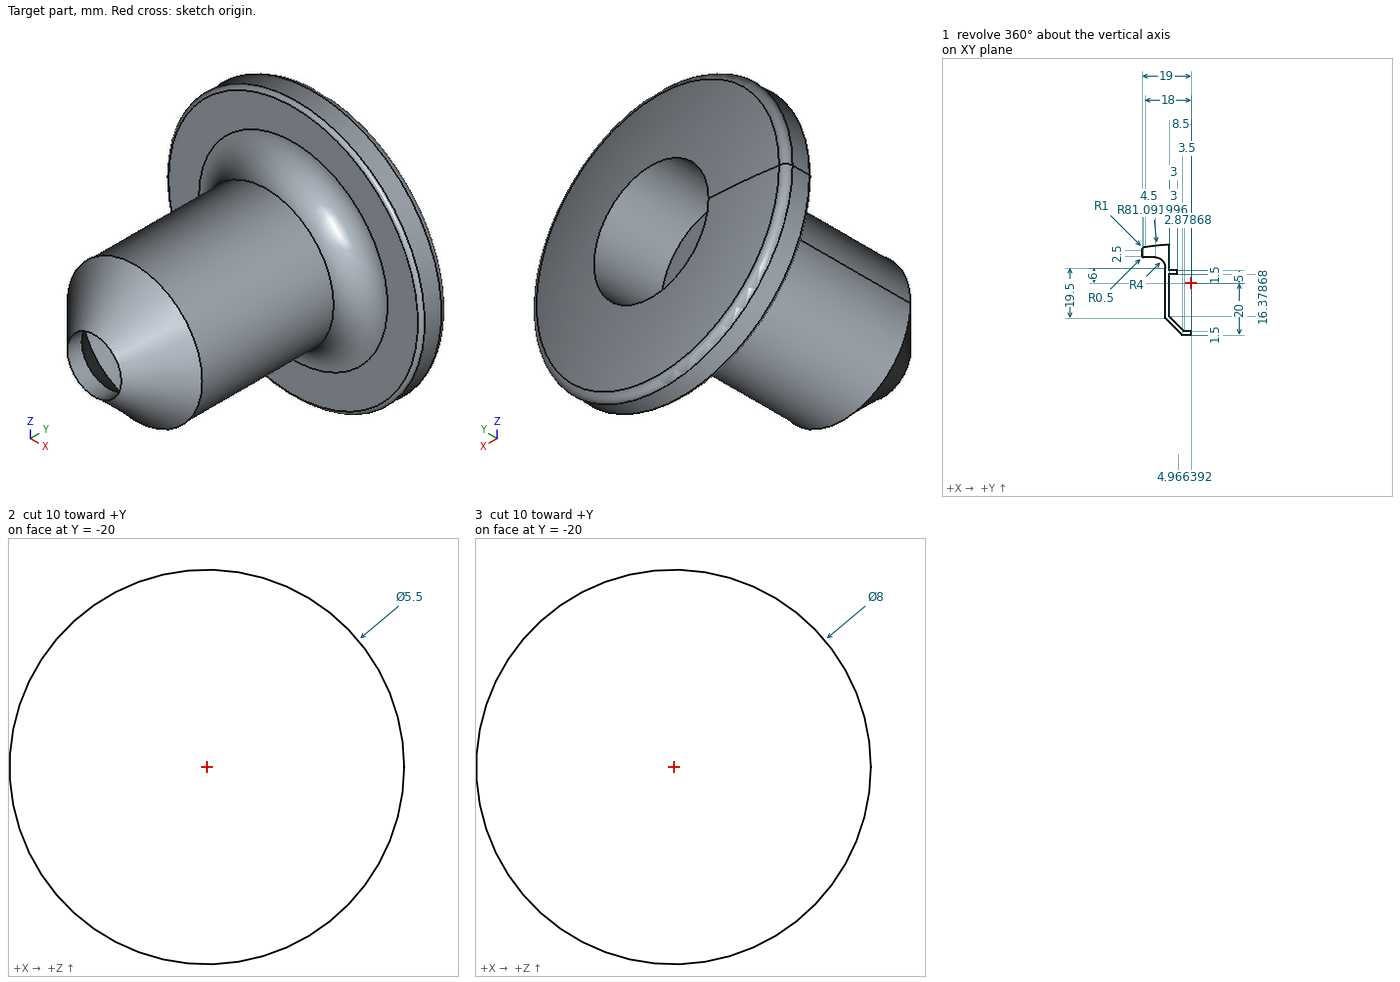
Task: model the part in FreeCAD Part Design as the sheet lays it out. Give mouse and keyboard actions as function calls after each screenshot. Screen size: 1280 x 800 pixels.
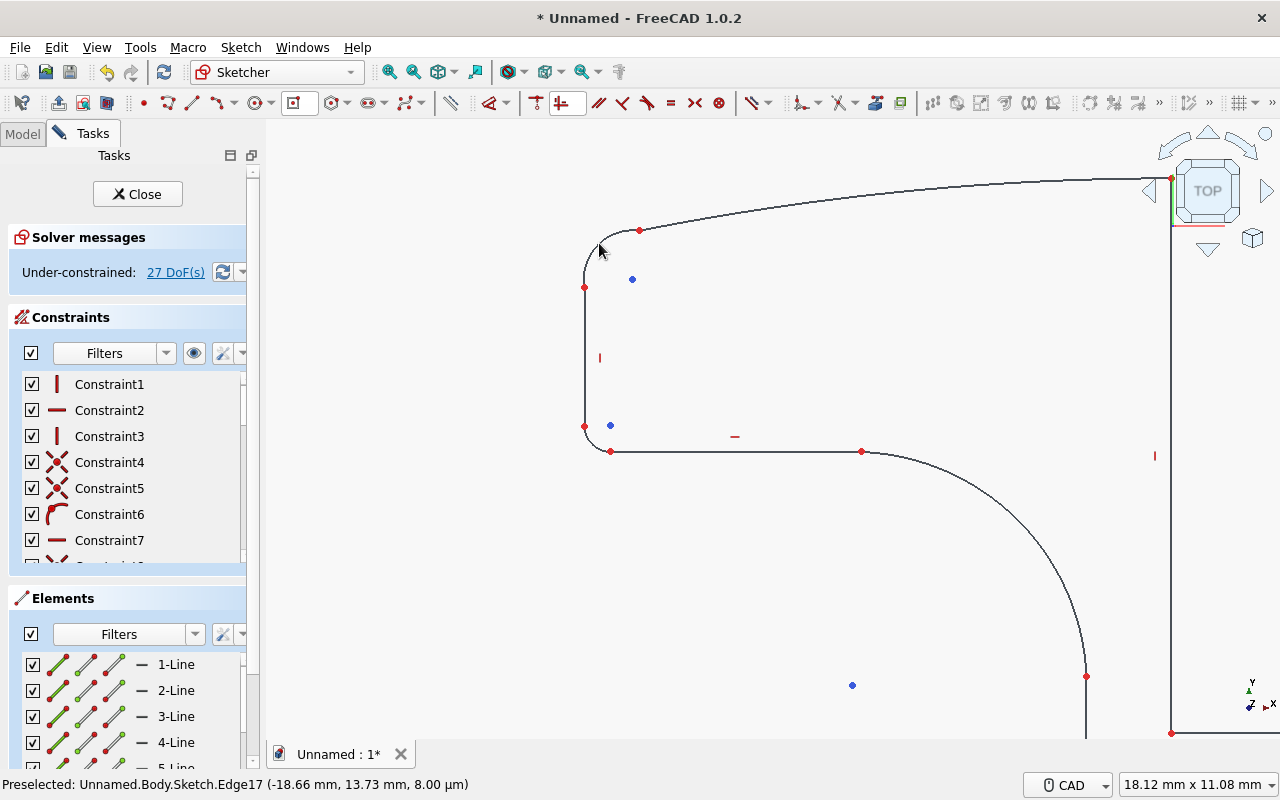
scroll(601, 247, down, 8)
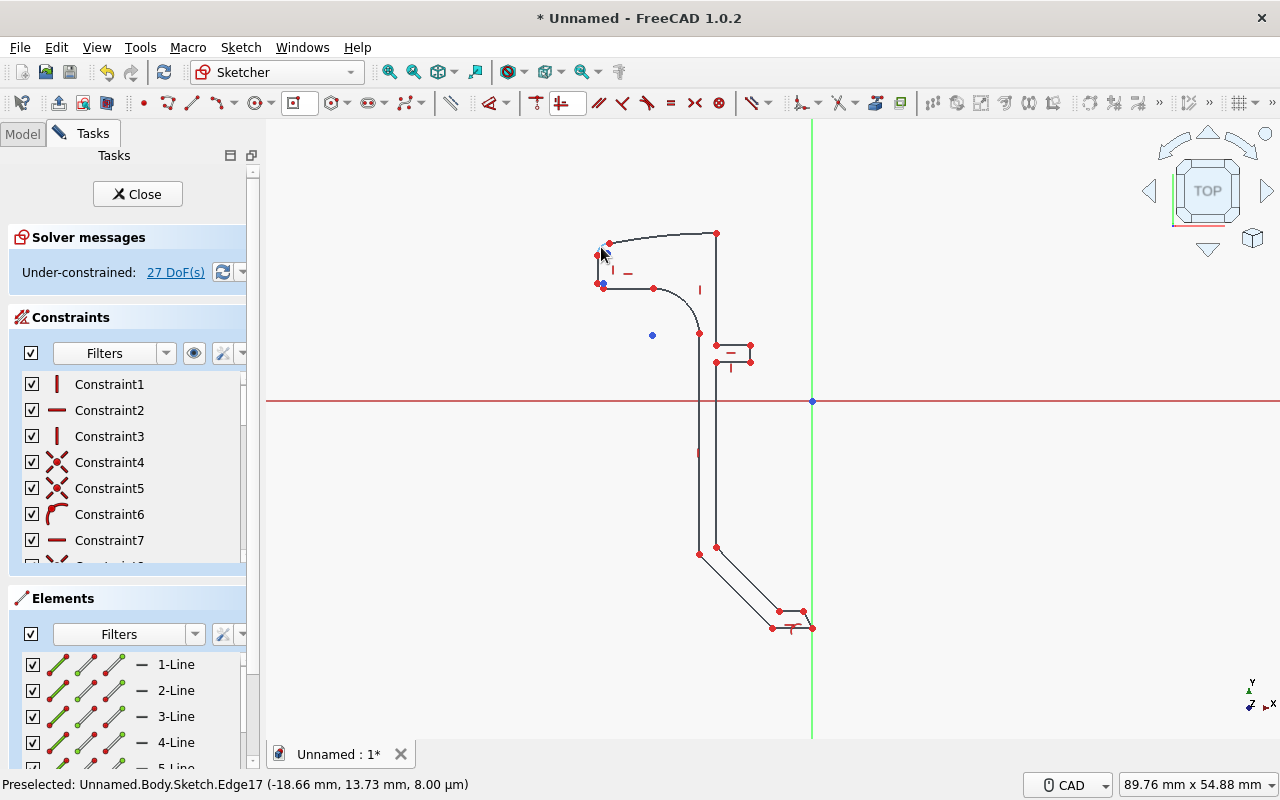
scroll(598, 264, up, 3)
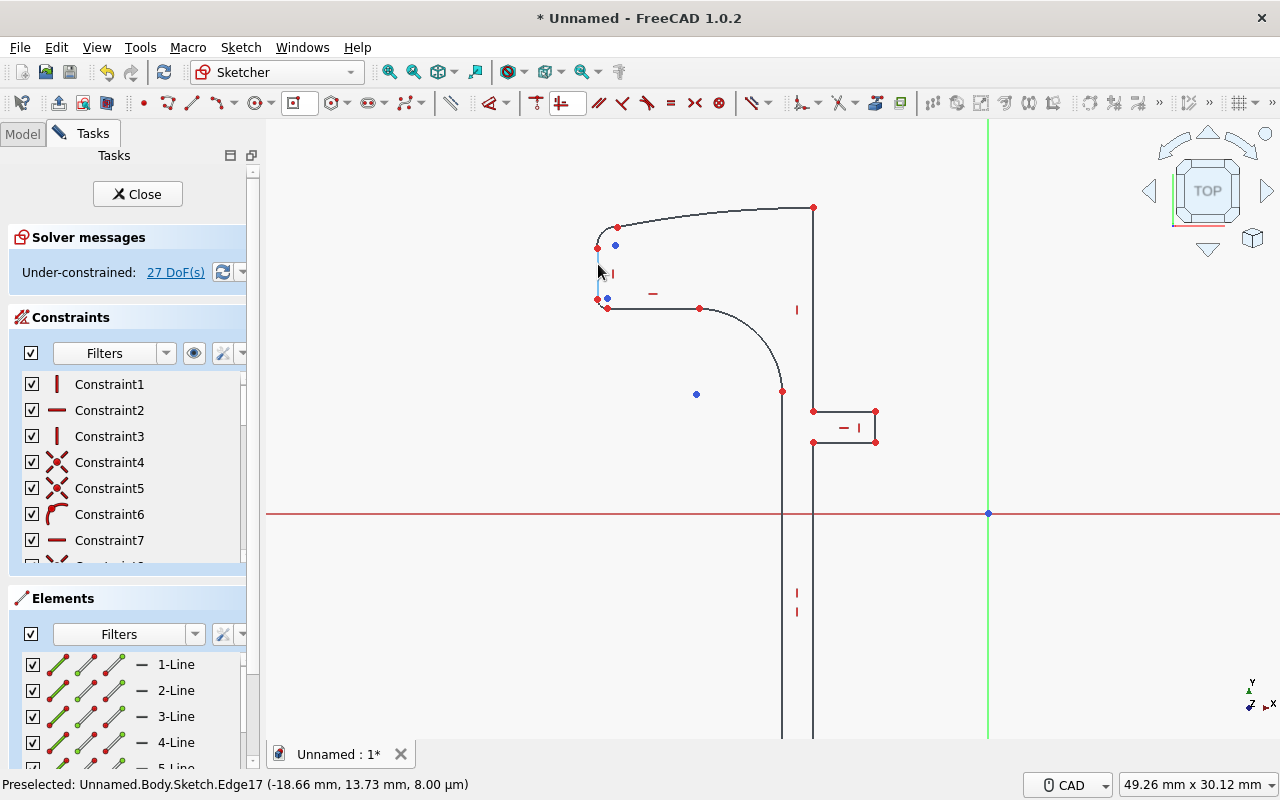
click(598, 263)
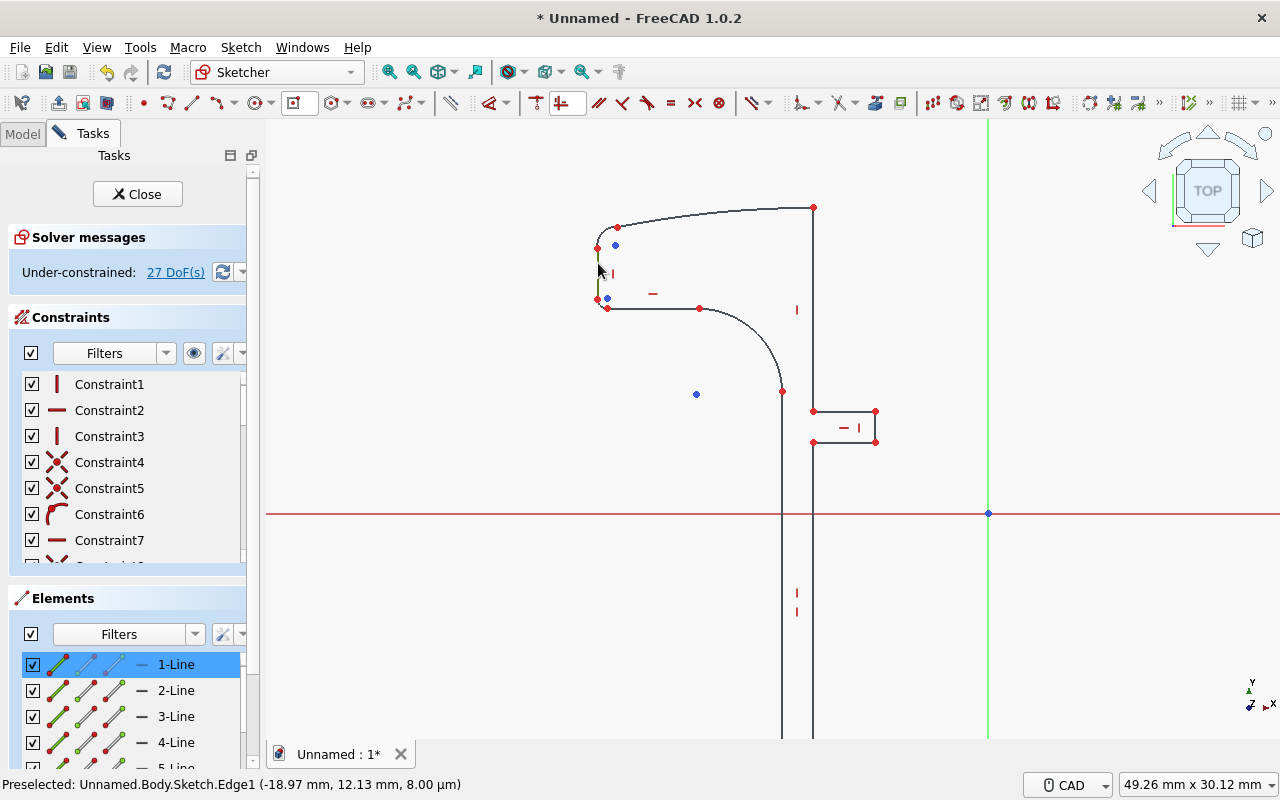
scroll(600, 306, up, 4)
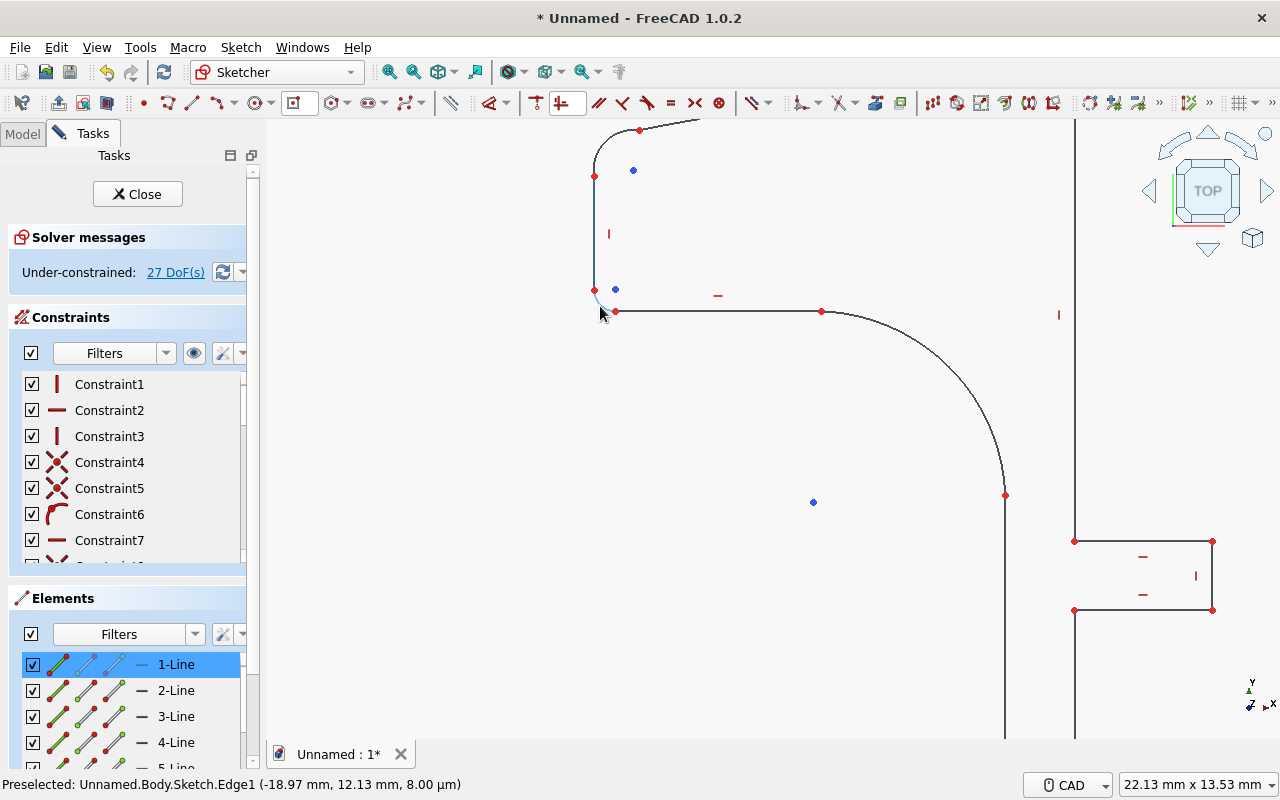
click(601, 305)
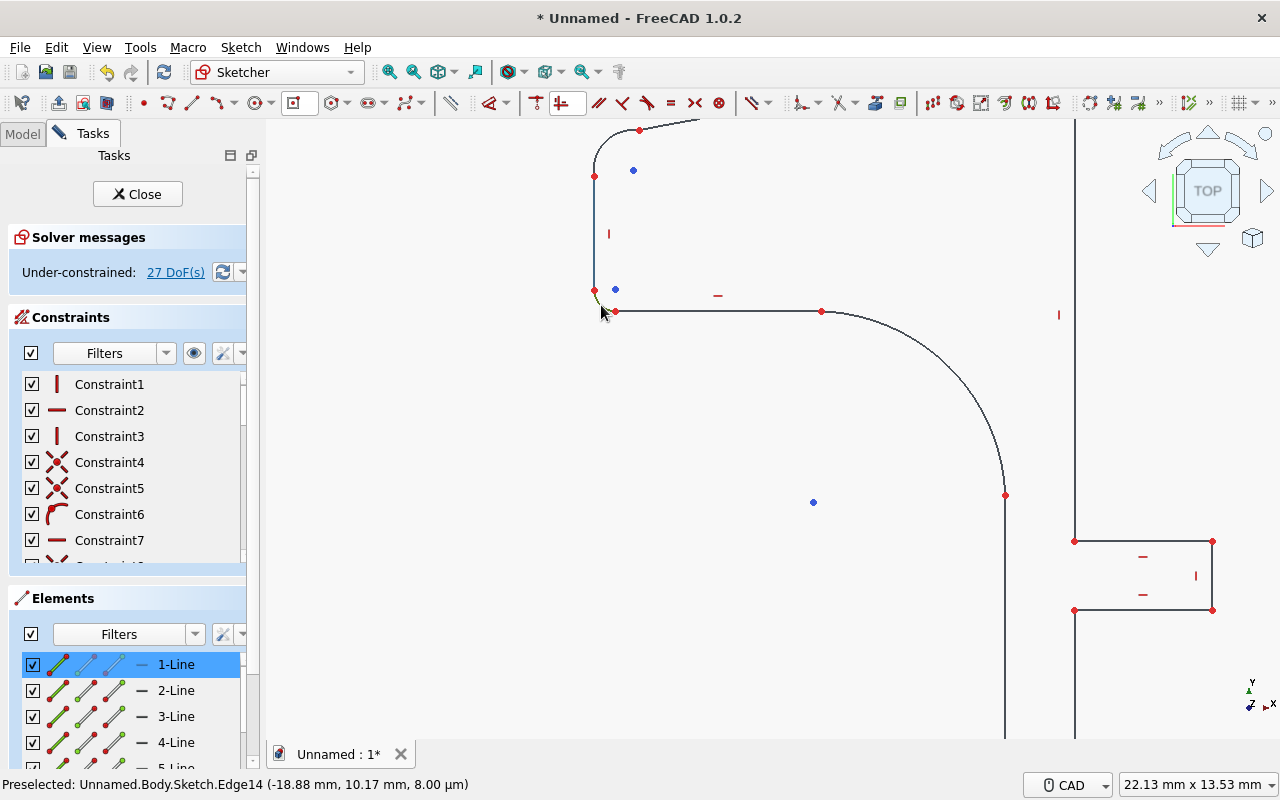
key(t)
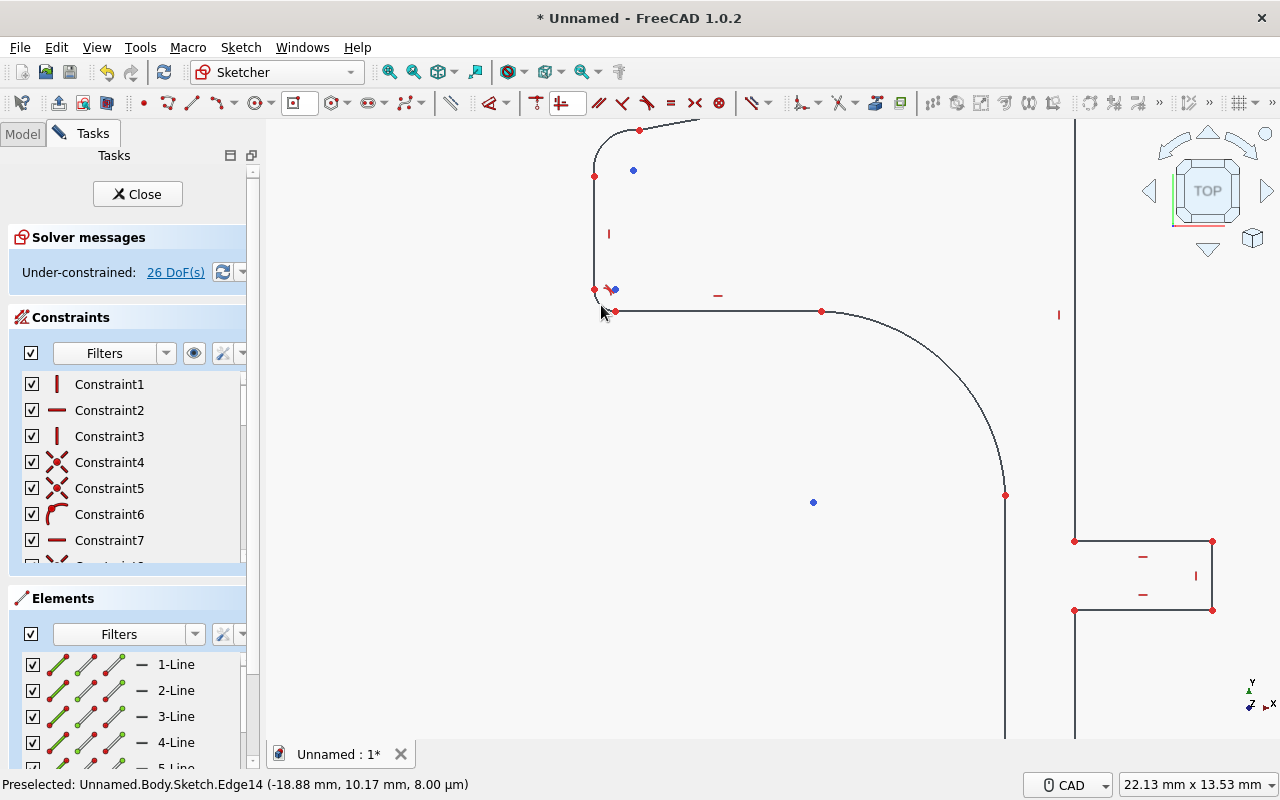
click(594, 211)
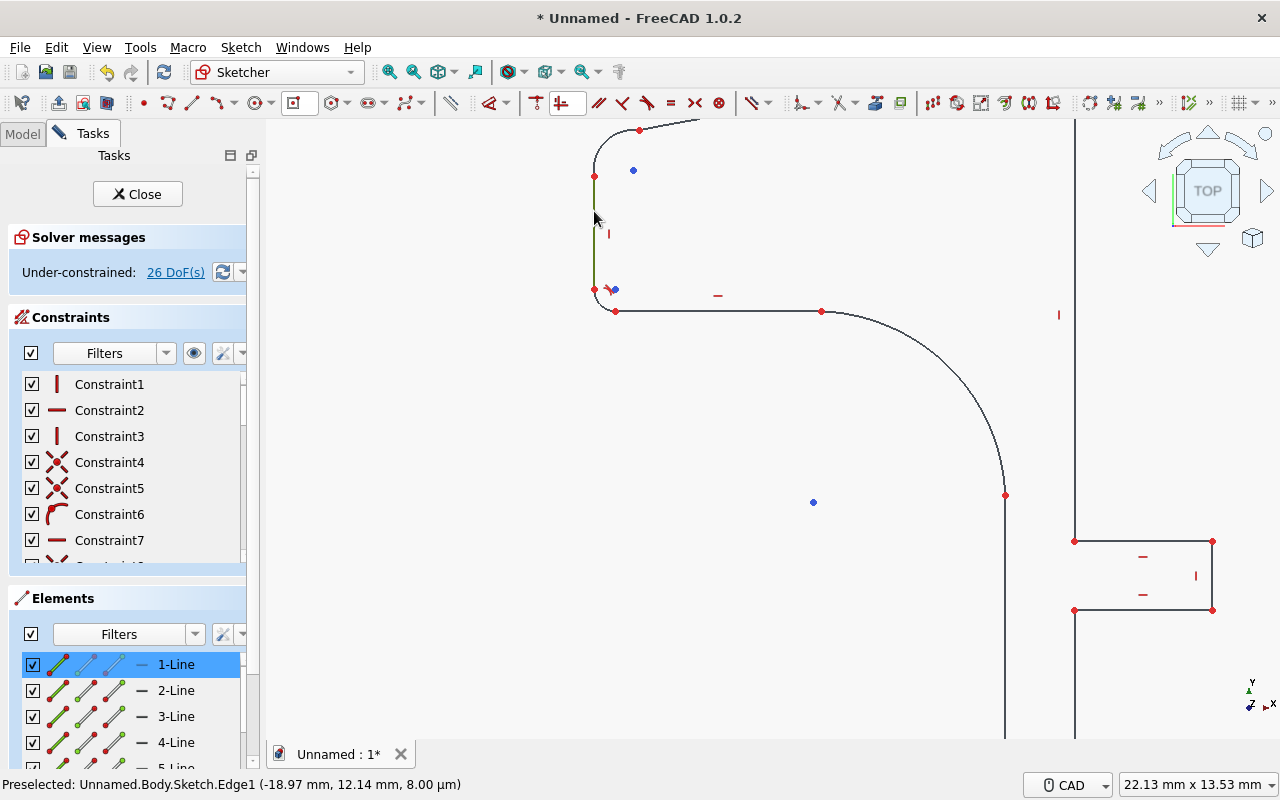
click(597, 155)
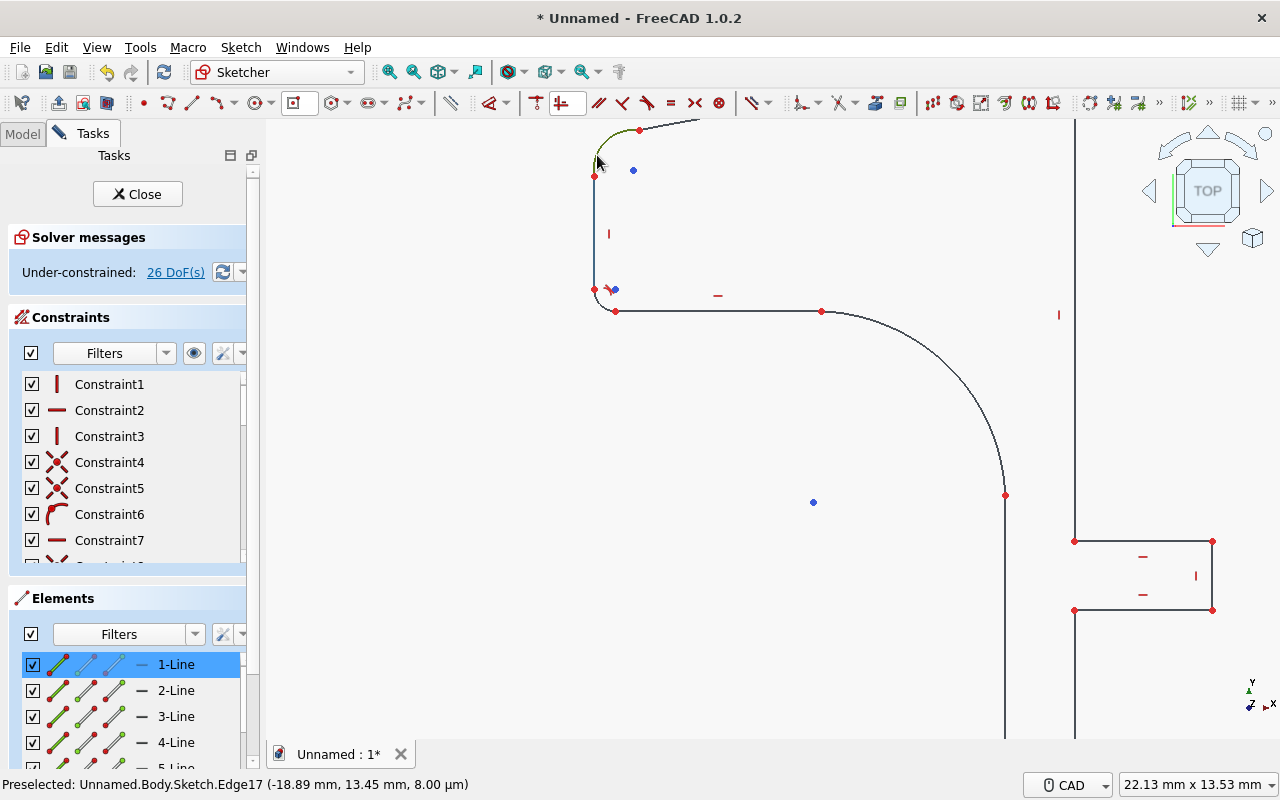
click(648, 104)